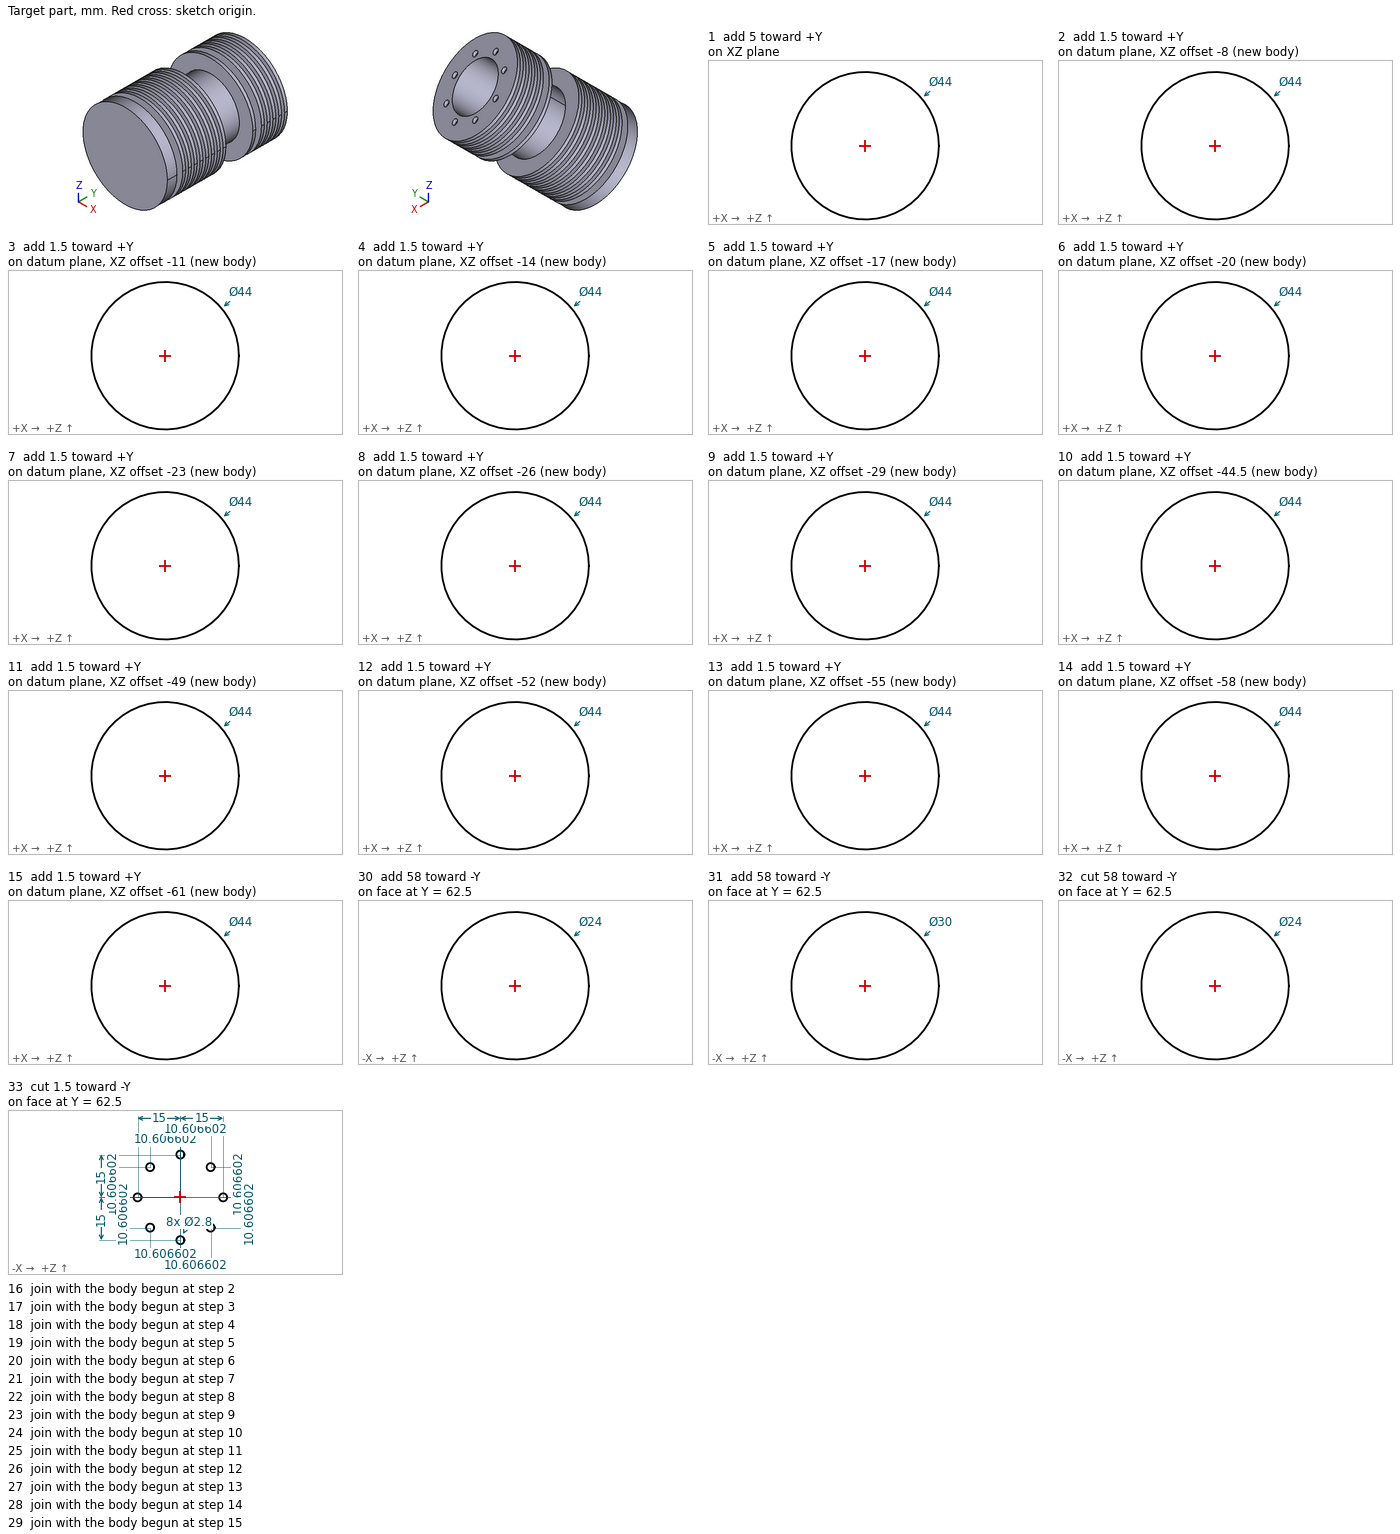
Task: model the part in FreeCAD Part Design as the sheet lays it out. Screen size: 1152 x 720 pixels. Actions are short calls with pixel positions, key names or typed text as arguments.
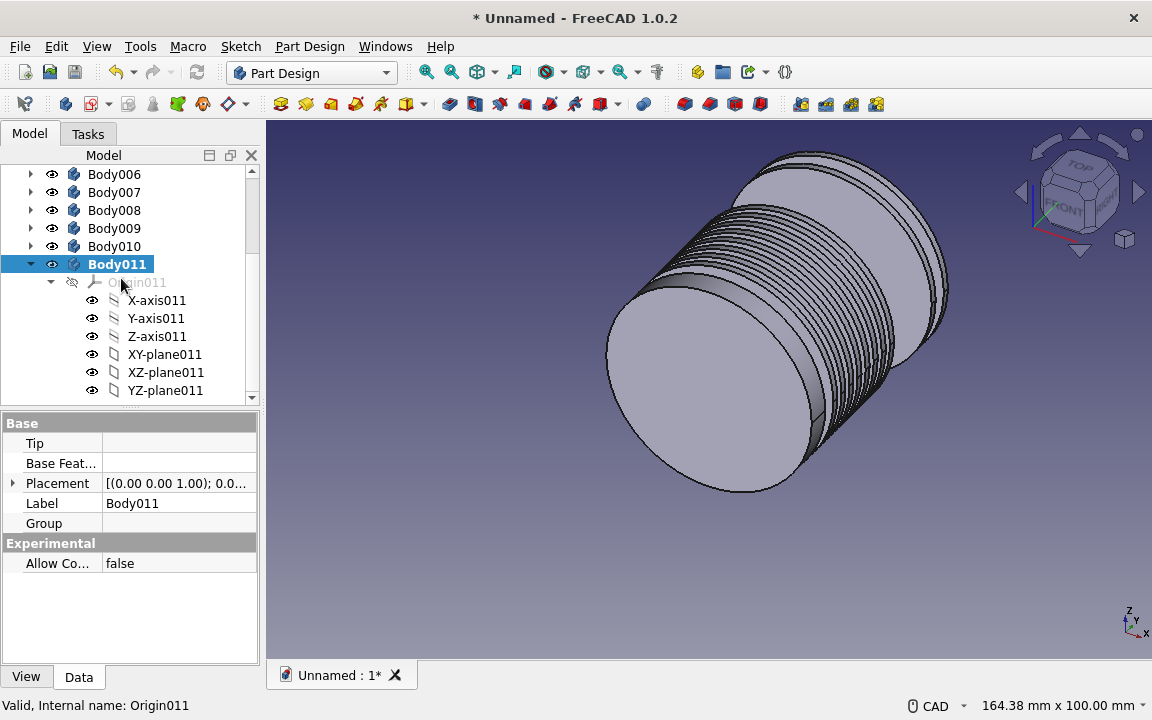
click(137, 372)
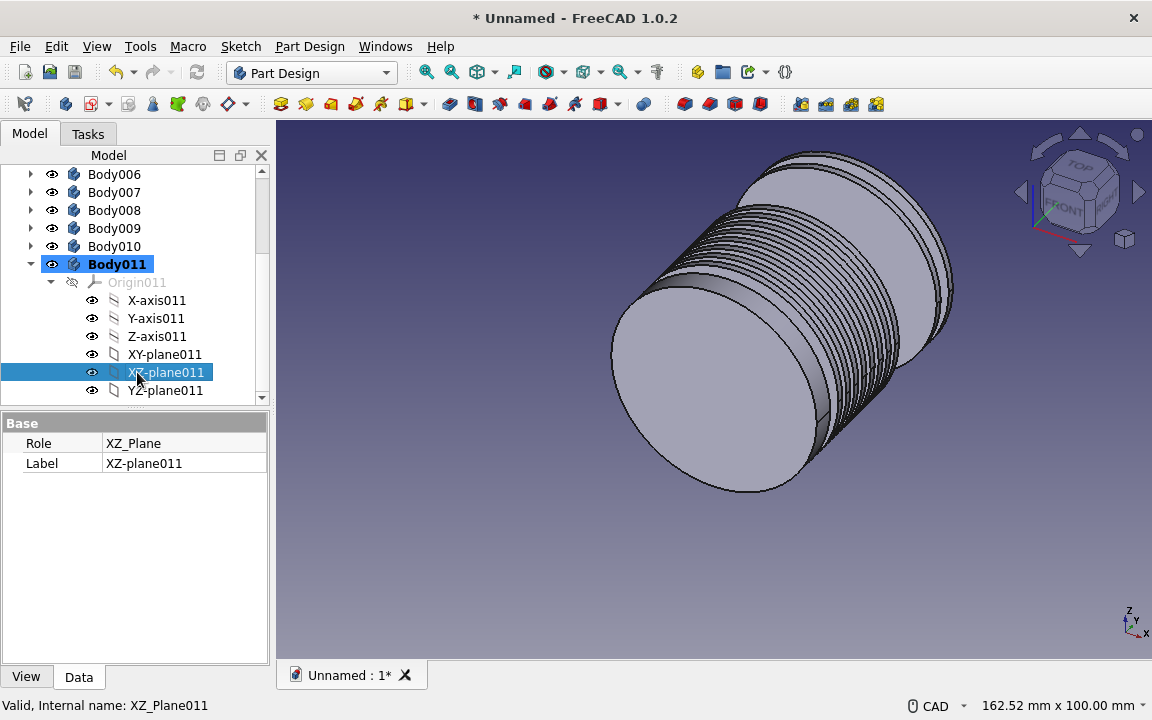
click(228, 104)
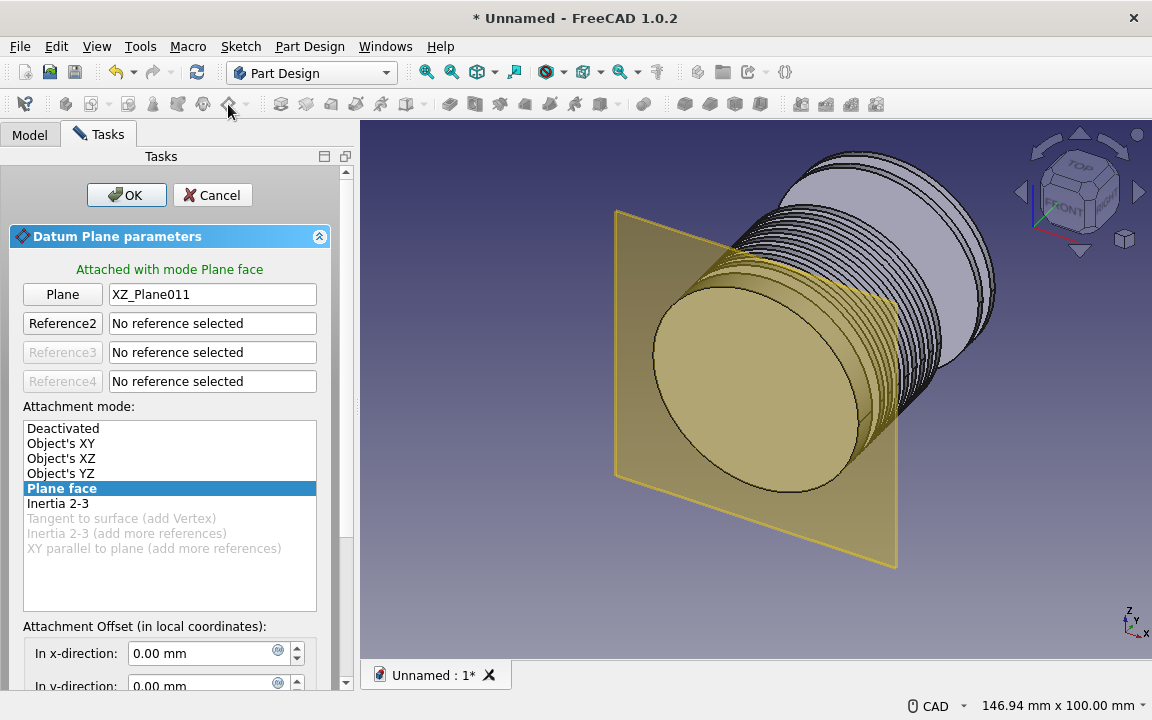
scroll(346, 428, down, 2)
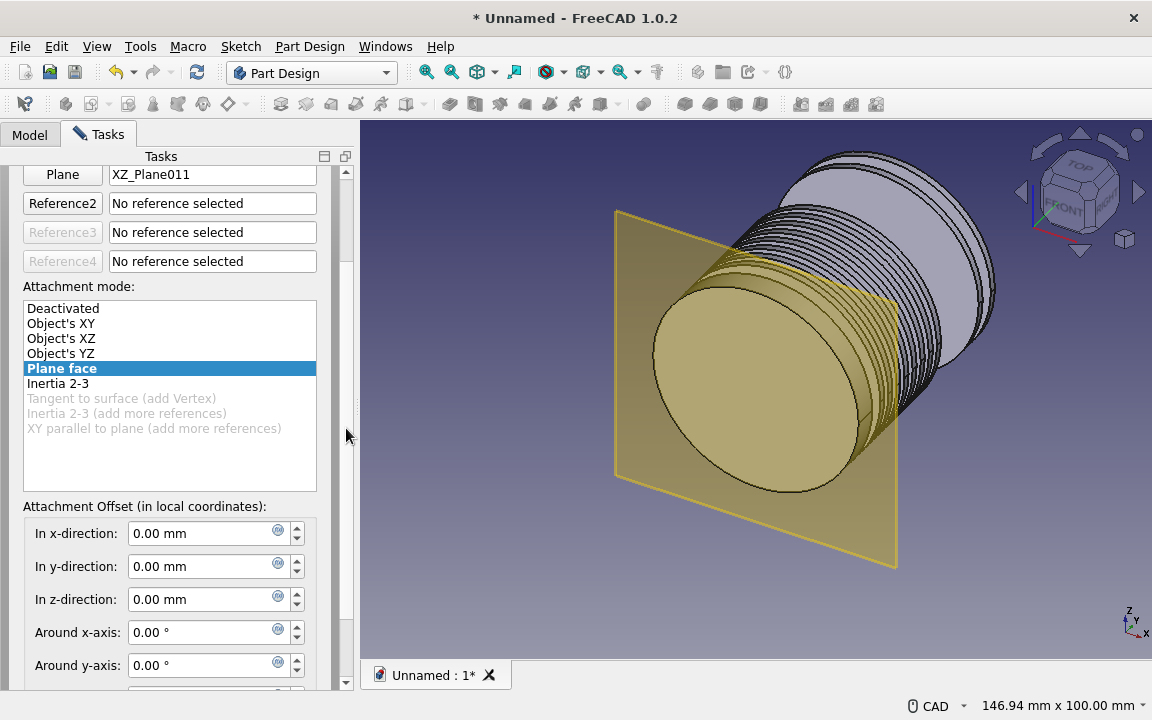
triple_click(210, 600)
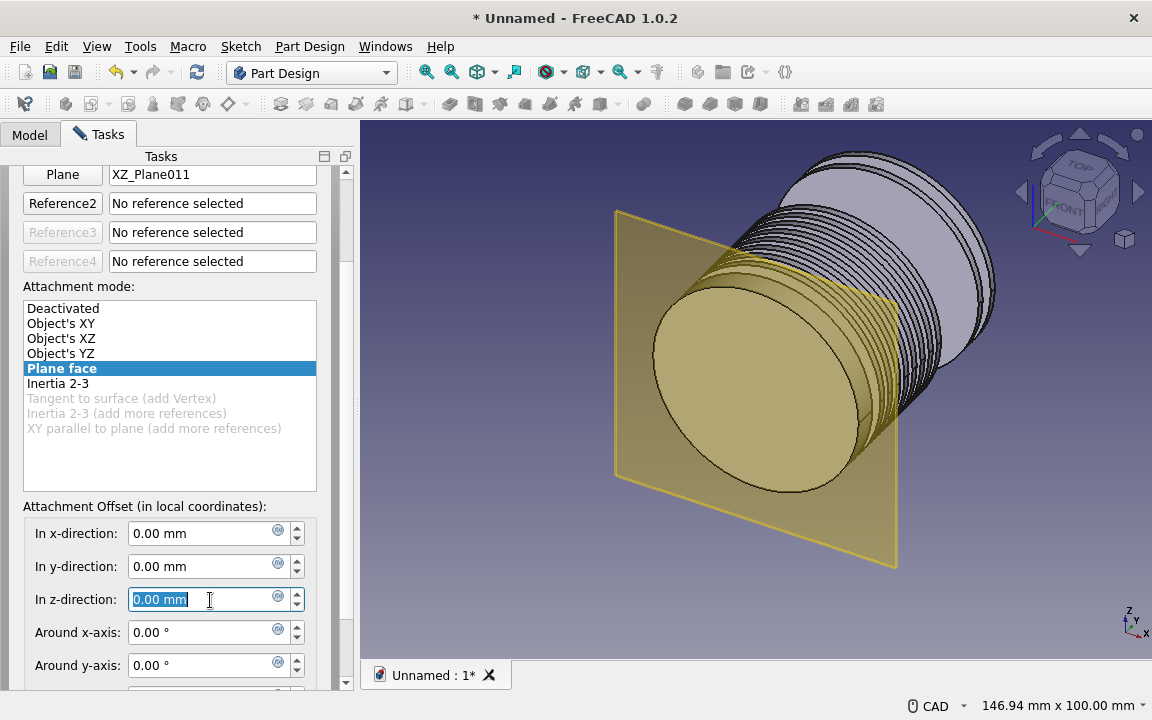
text(-52)
key(Tab)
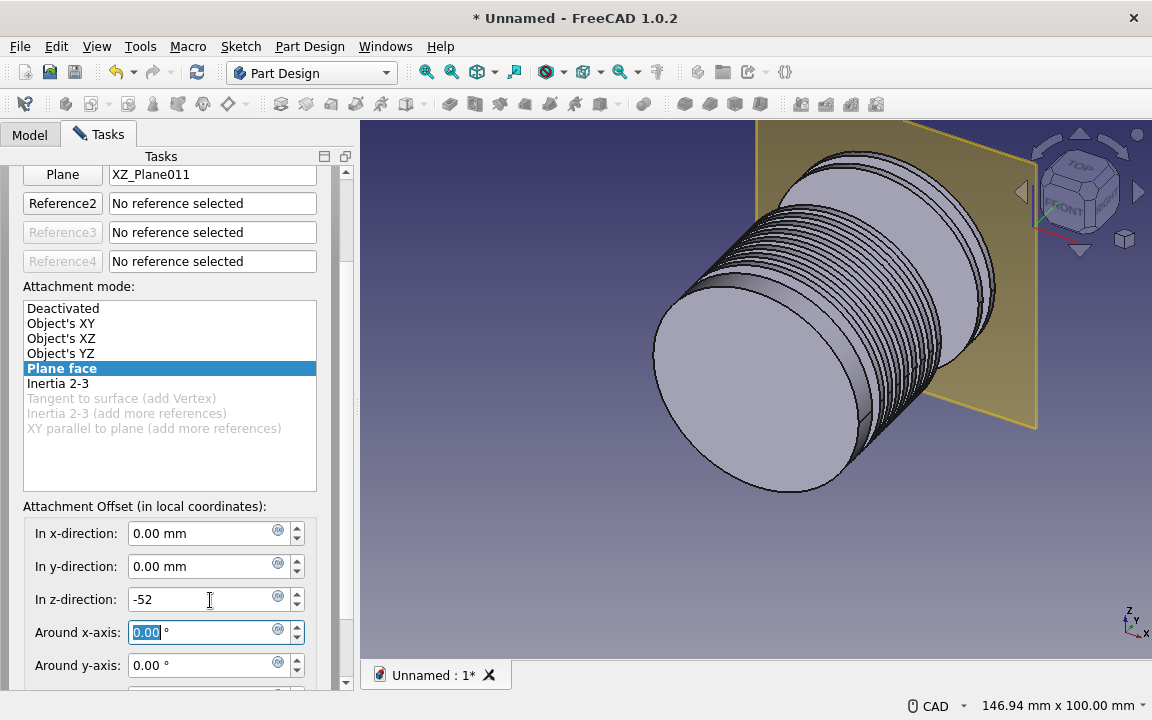
scroll(346, 428, up, 3)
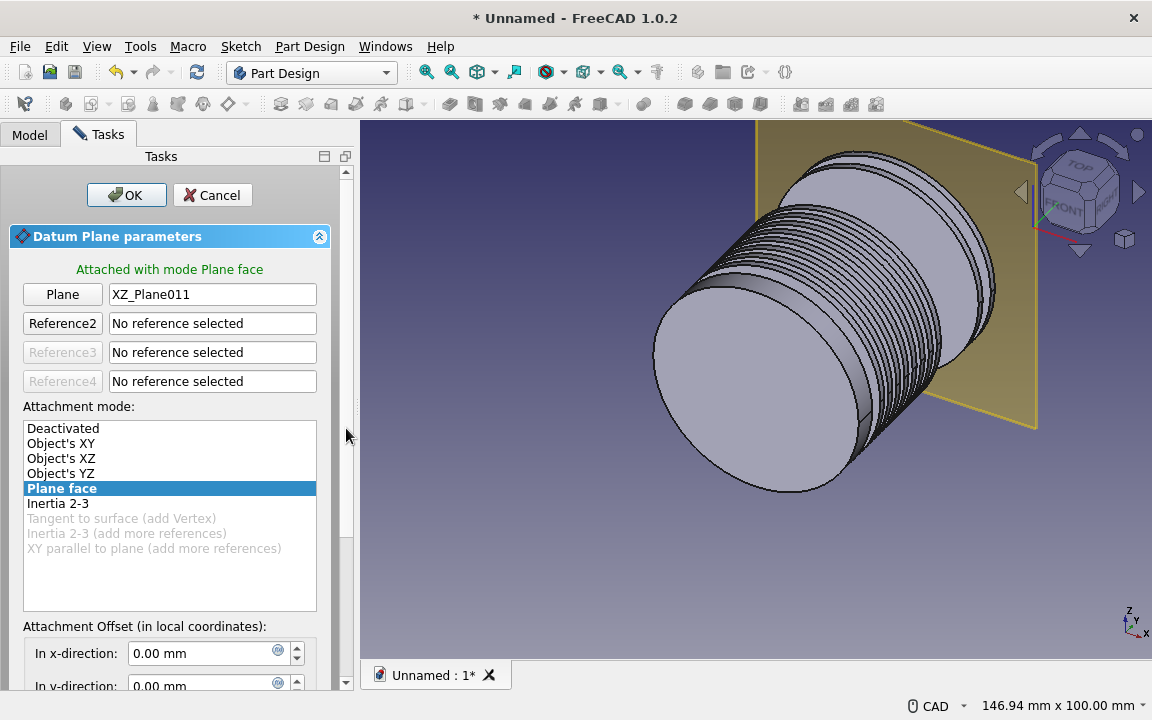
click(127, 195)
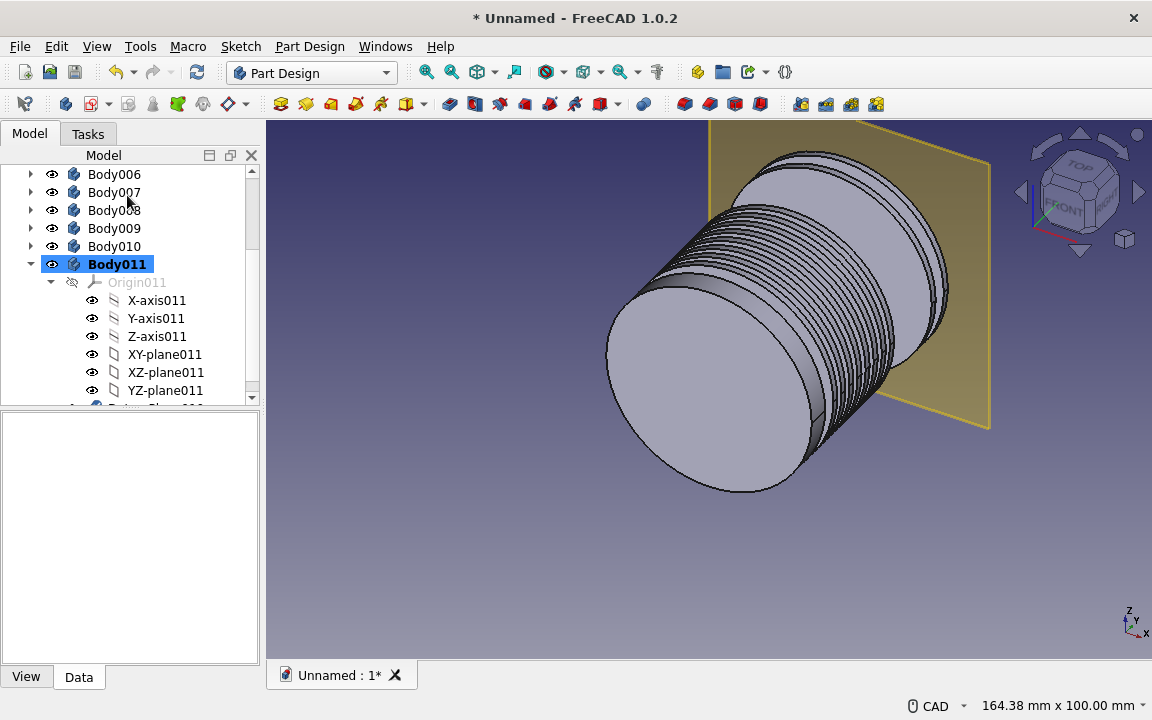
scroll(121, 278, down, 3)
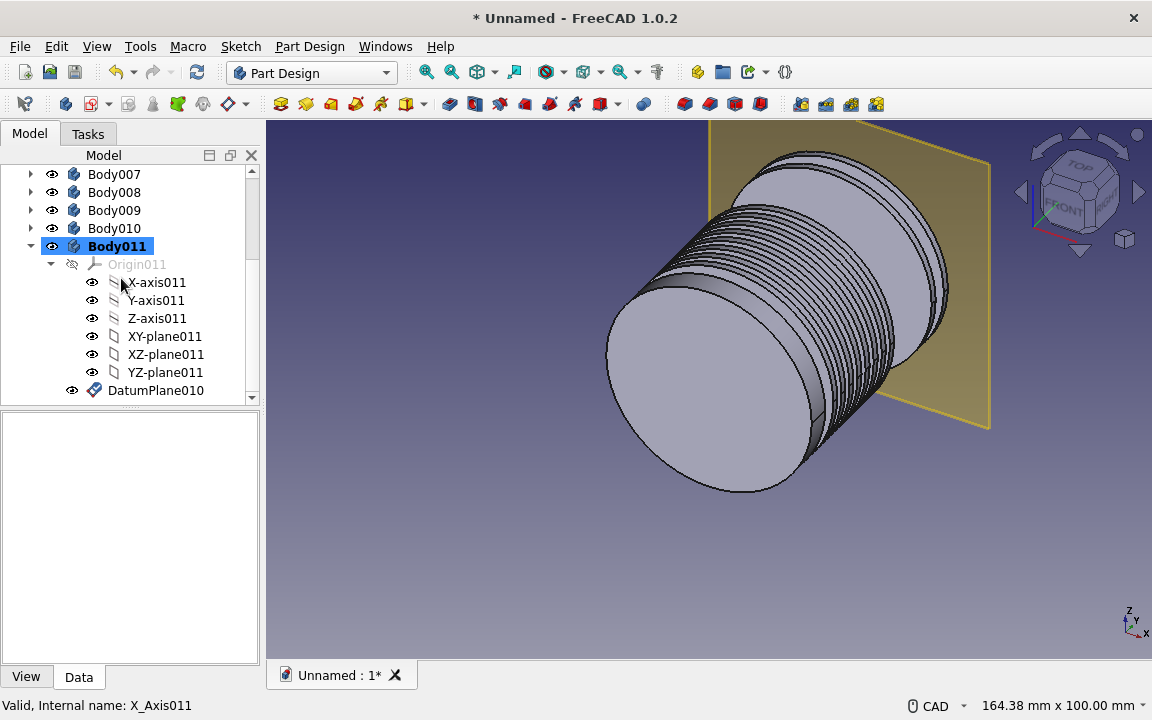
click(117, 390)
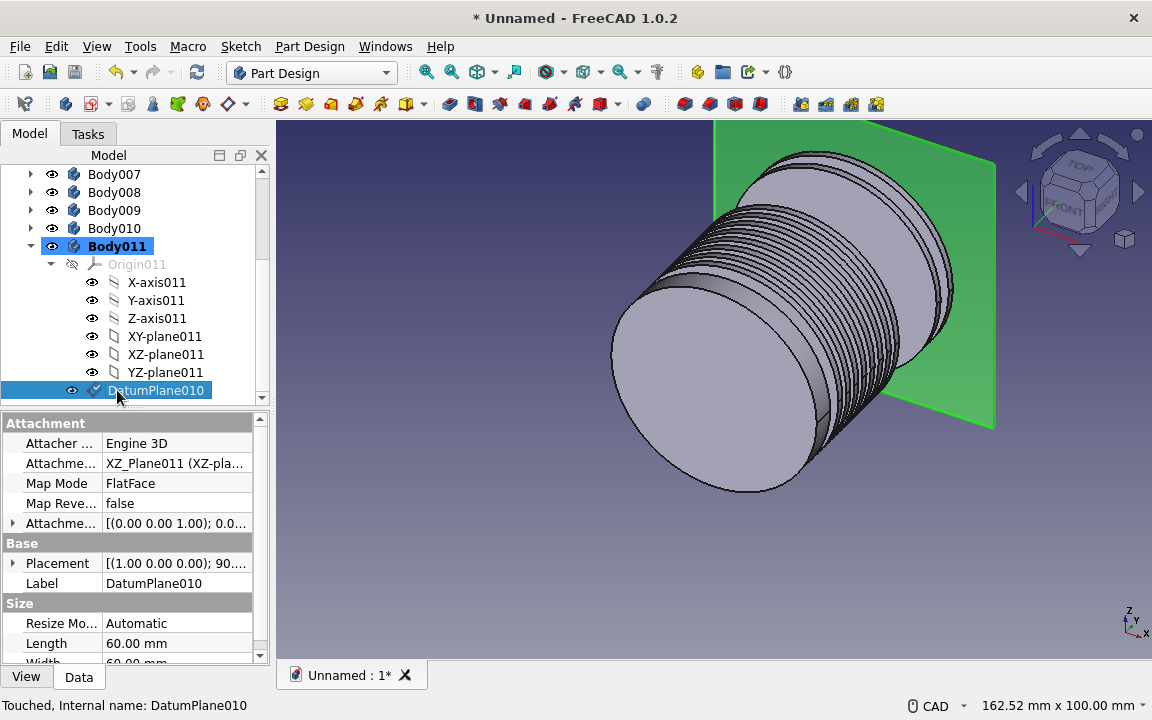
click(90, 104)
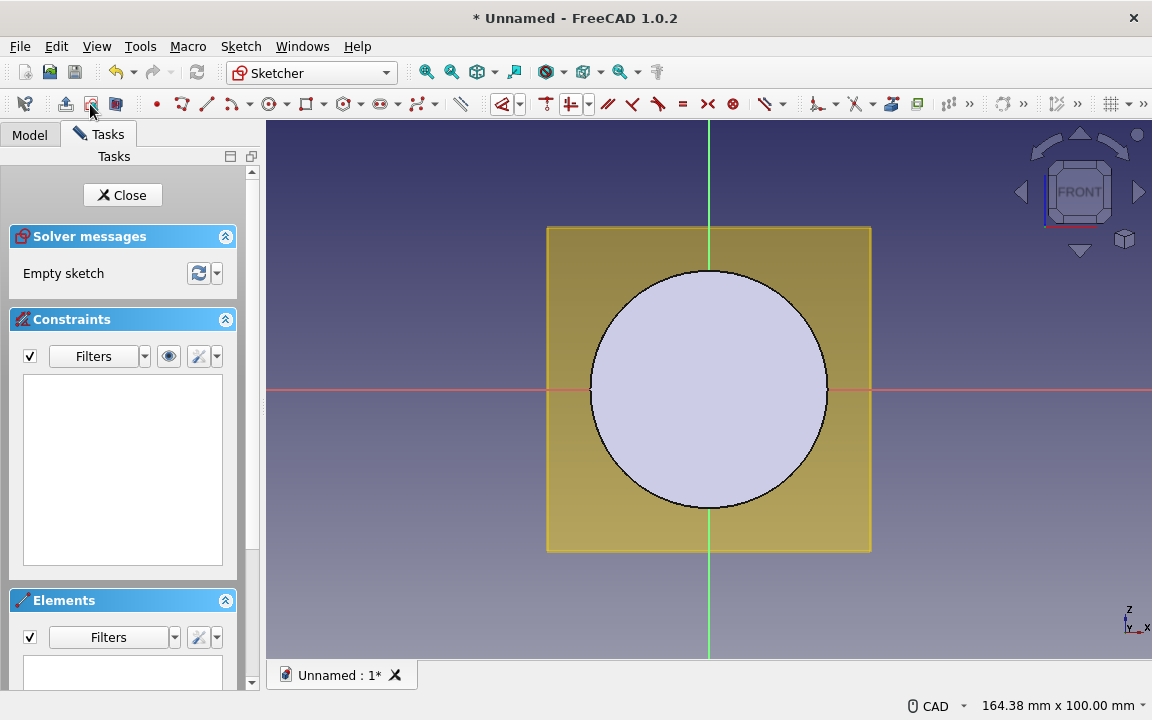
scroll(848, 390, up, 2)